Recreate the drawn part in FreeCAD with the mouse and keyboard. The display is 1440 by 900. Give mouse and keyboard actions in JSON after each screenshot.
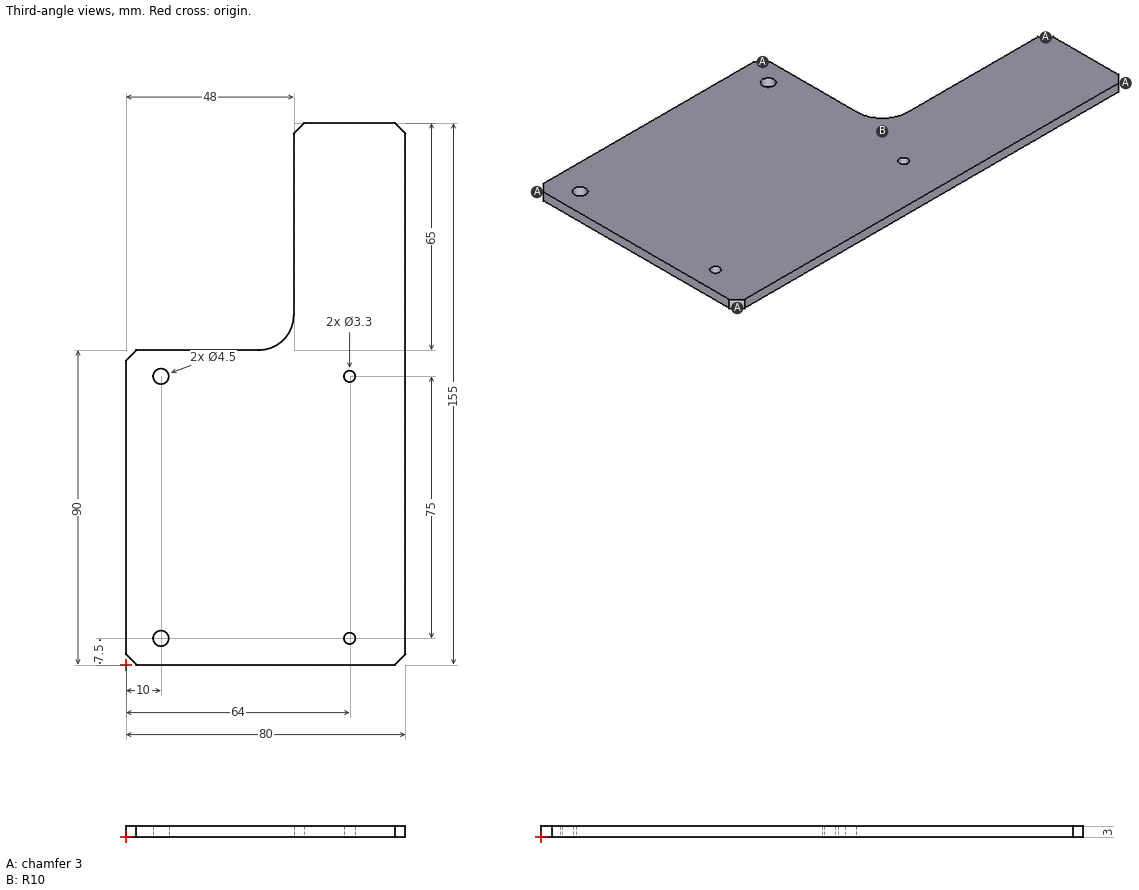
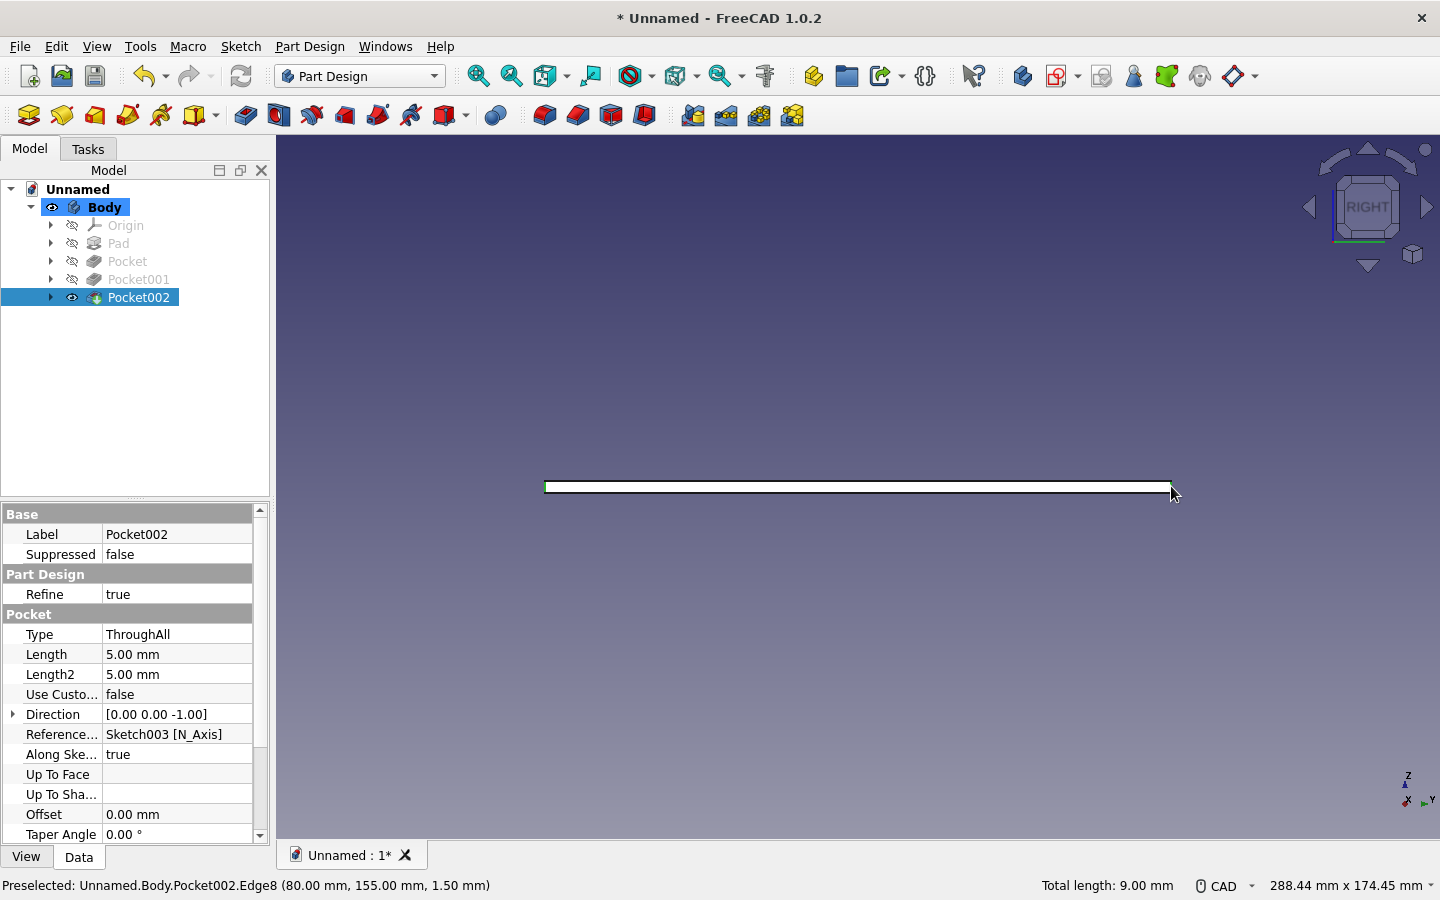
{"action": "scroll", "coordinate": [1171, 486], "scroll_direction": "up", "scroll_amount": 6}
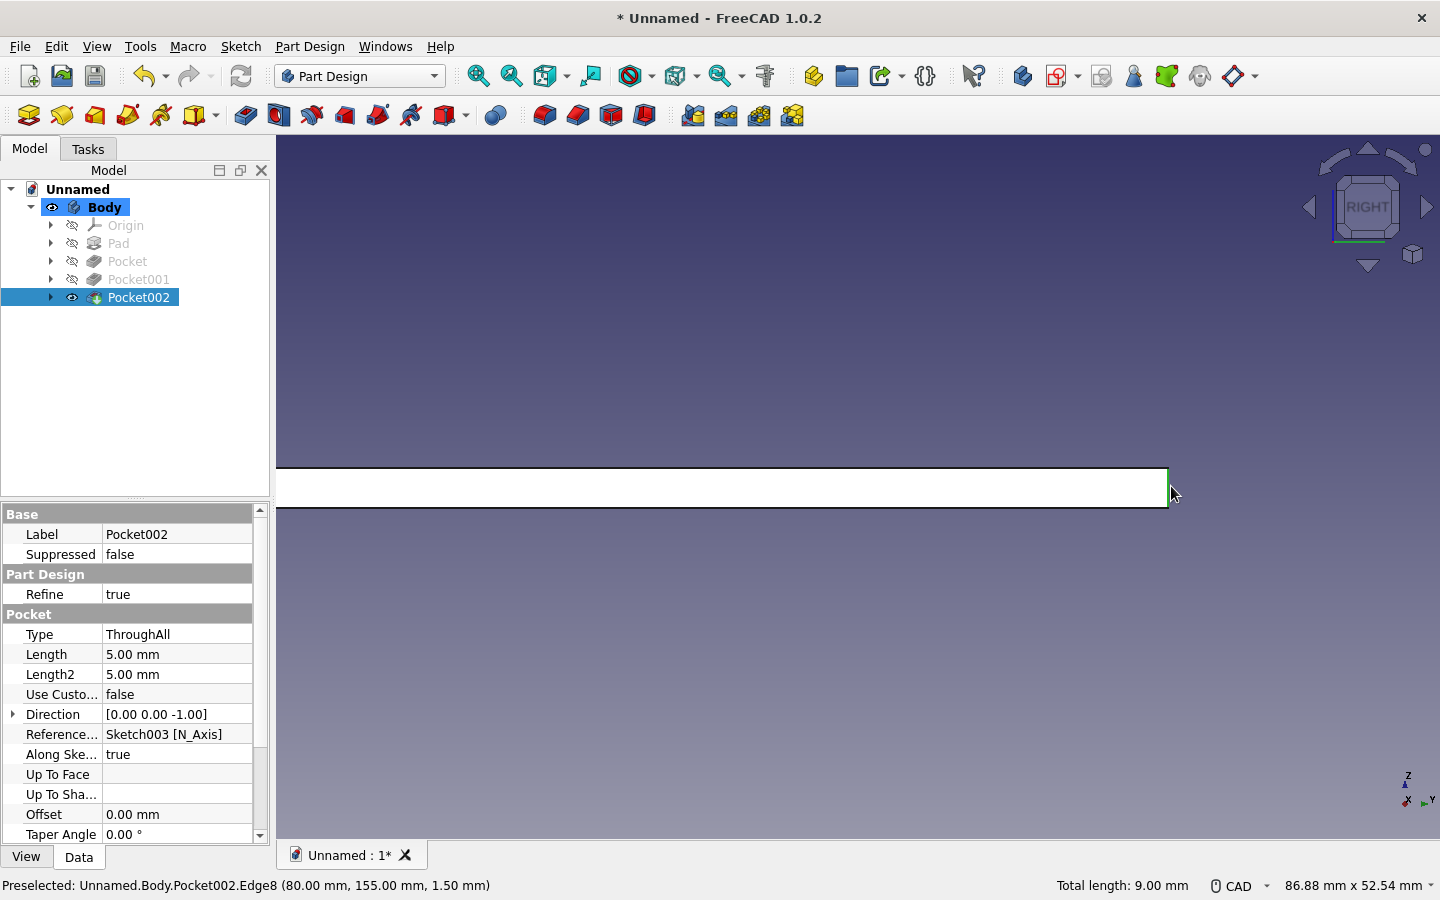
{"action": "key", "text": "v f"}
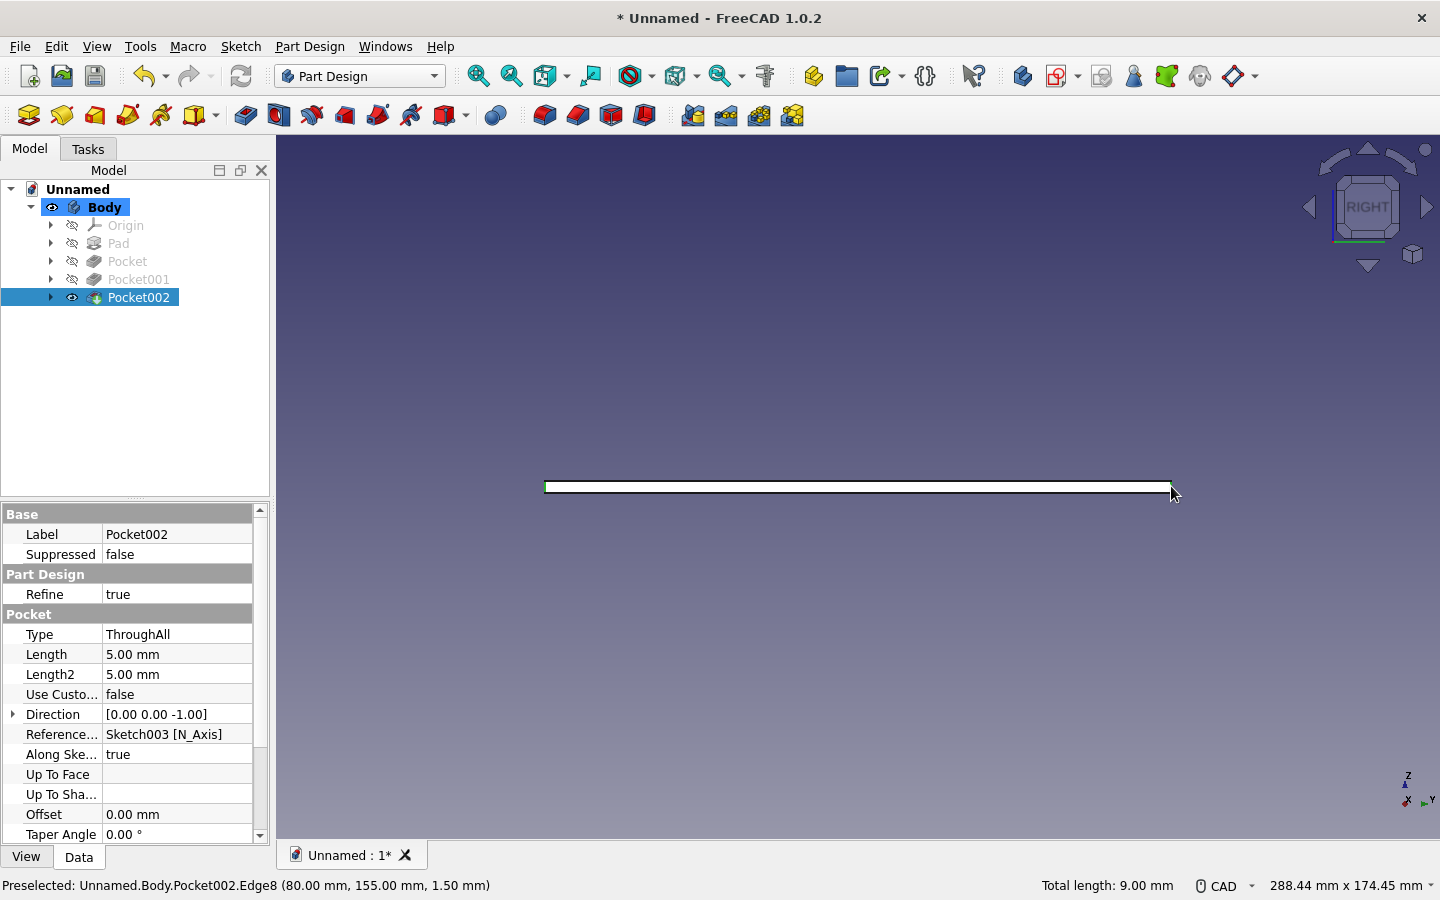
{"action": "key", "text": "5"}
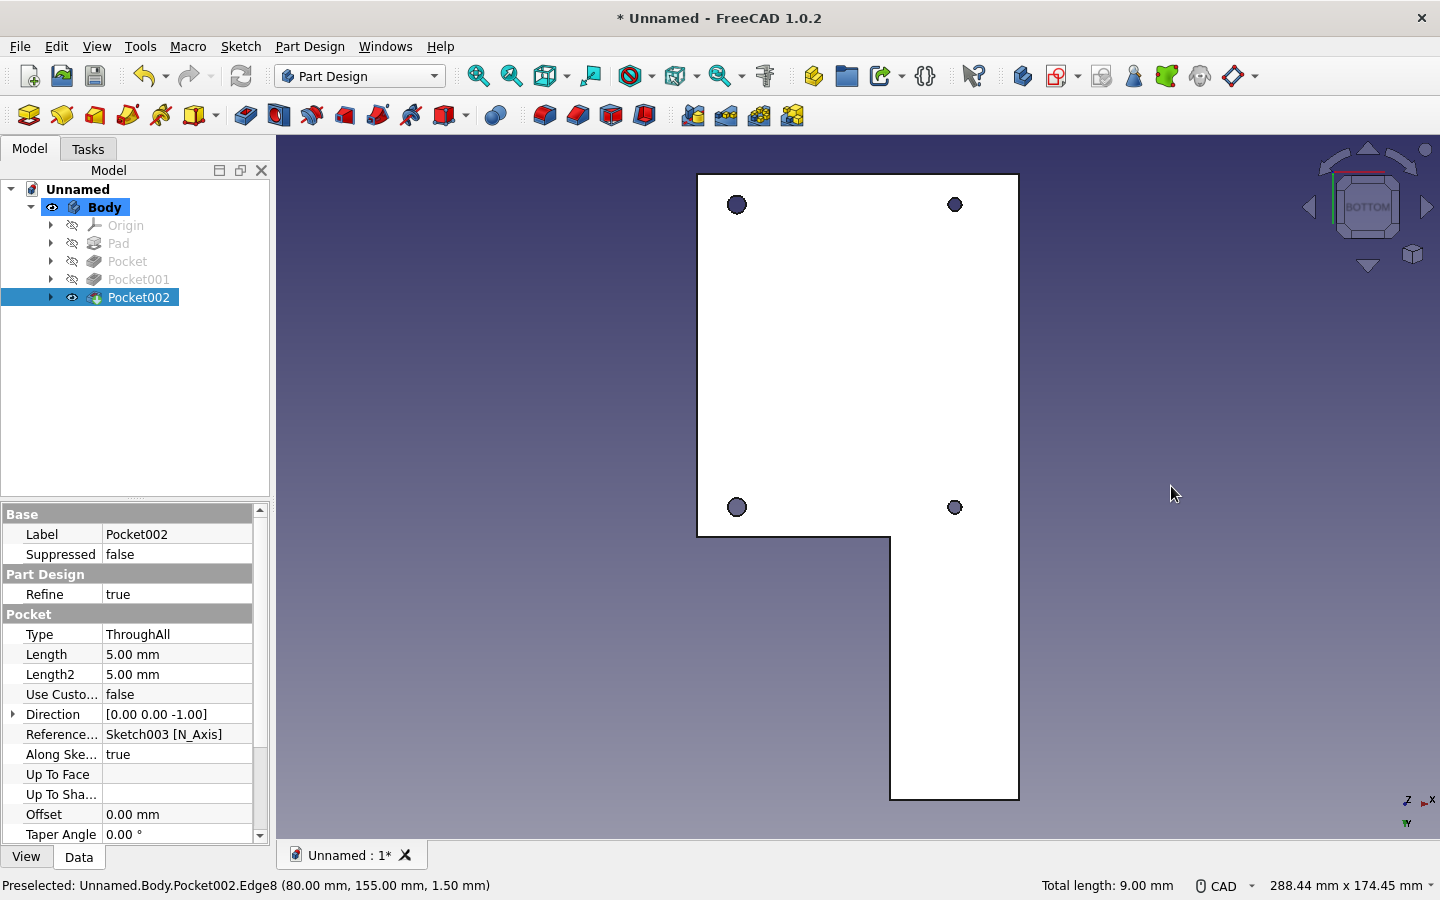
{"action": "scroll", "coordinate": [890, 799], "scroll_direction": "up", "scroll_amount": 6}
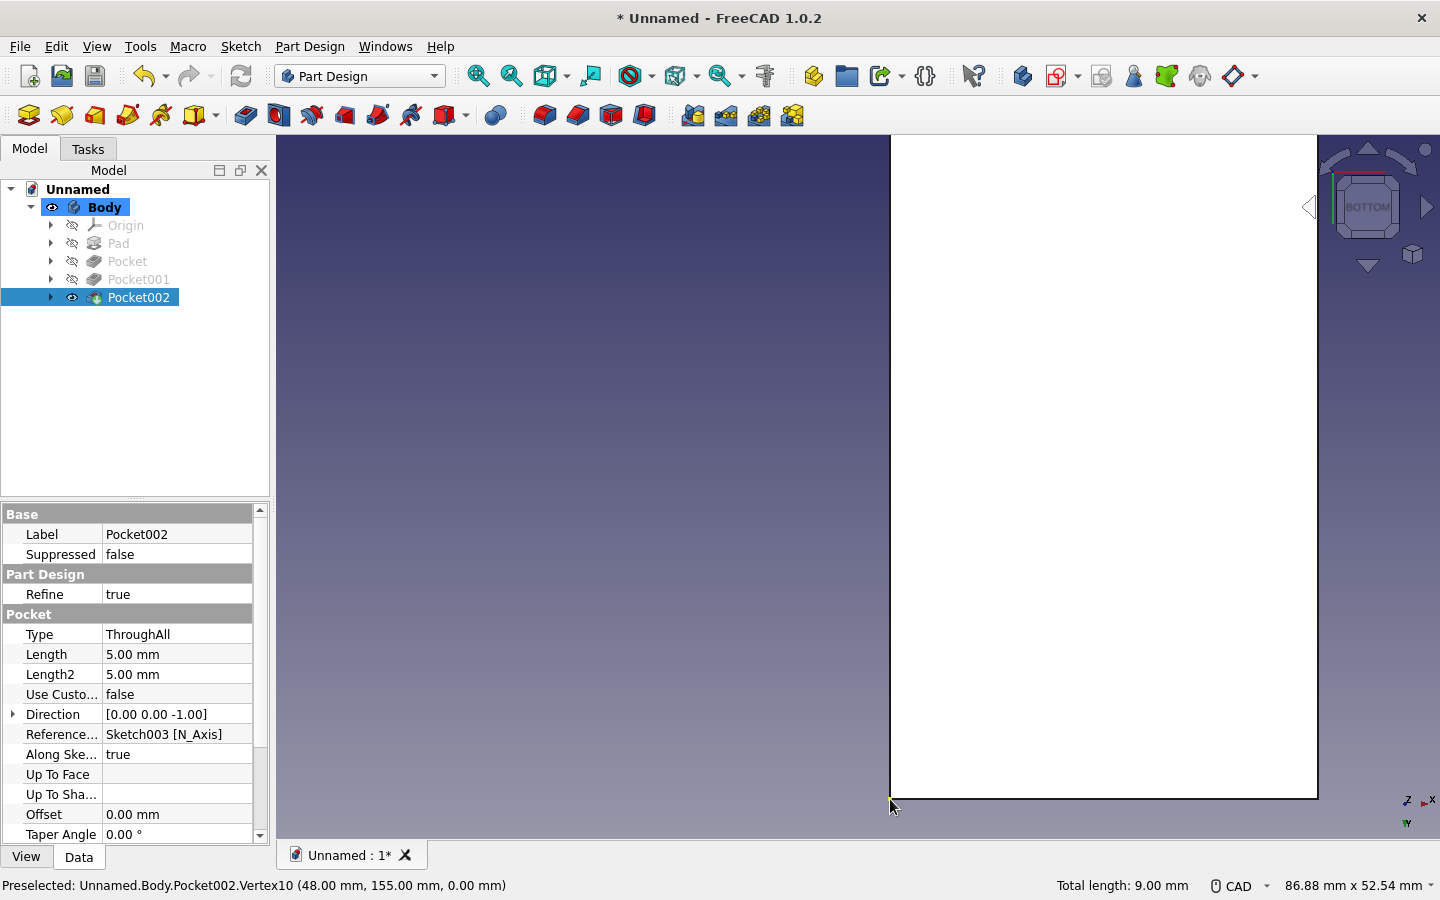
{"action": "key", "text": "v f"}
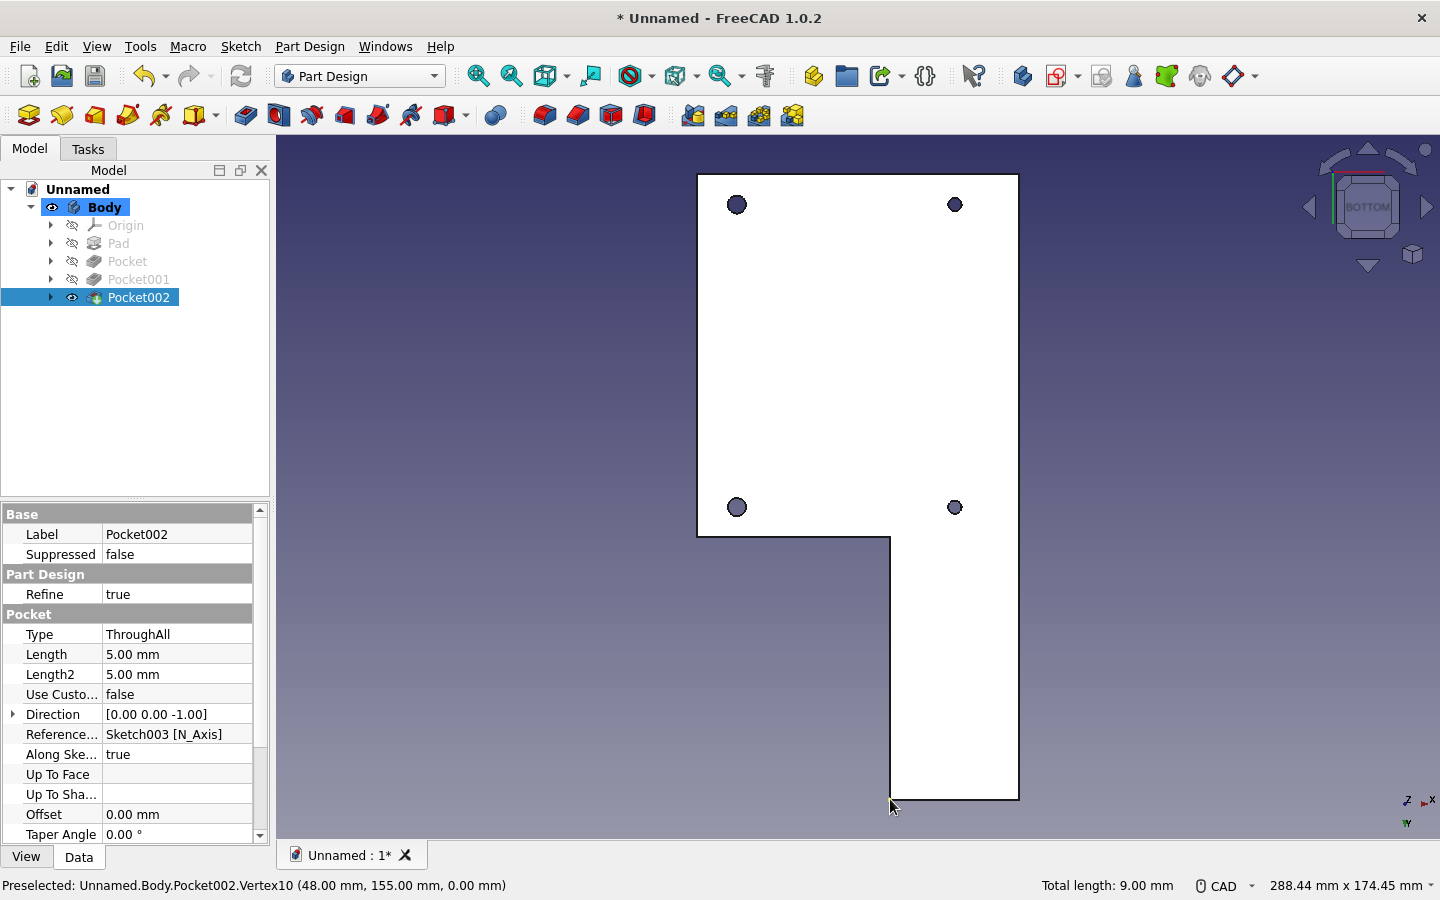
{"action": "key", "text": "4"}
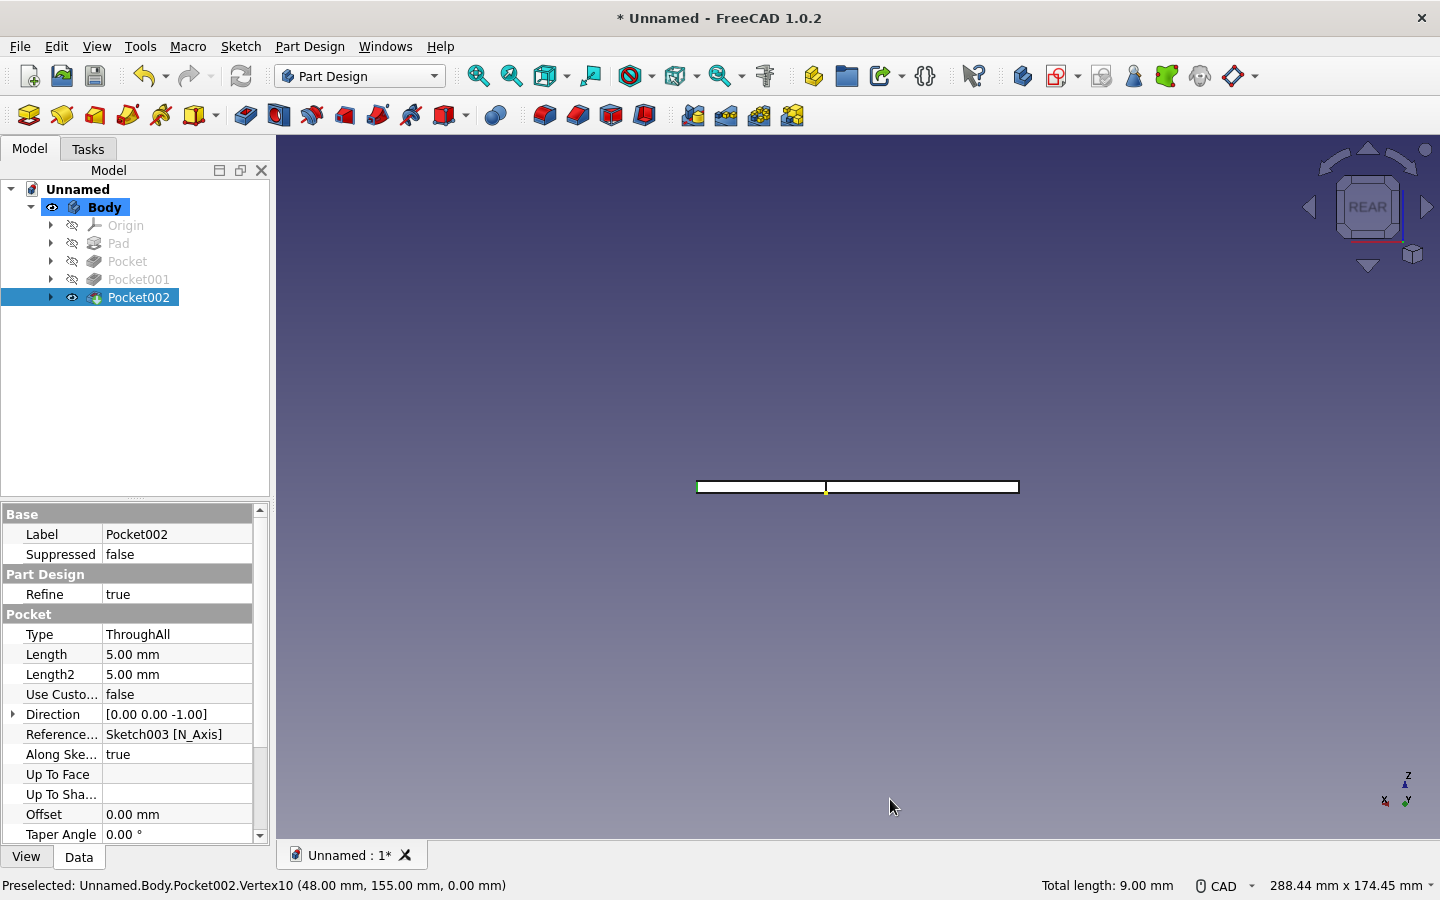
{"action": "left_click", "coordinate": [479, 76]}